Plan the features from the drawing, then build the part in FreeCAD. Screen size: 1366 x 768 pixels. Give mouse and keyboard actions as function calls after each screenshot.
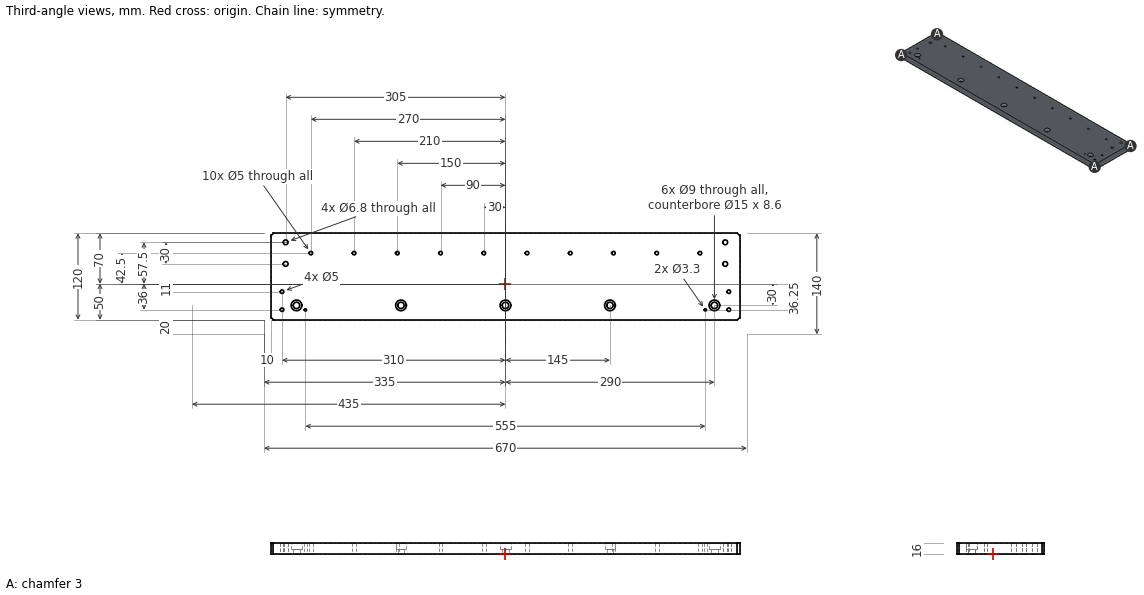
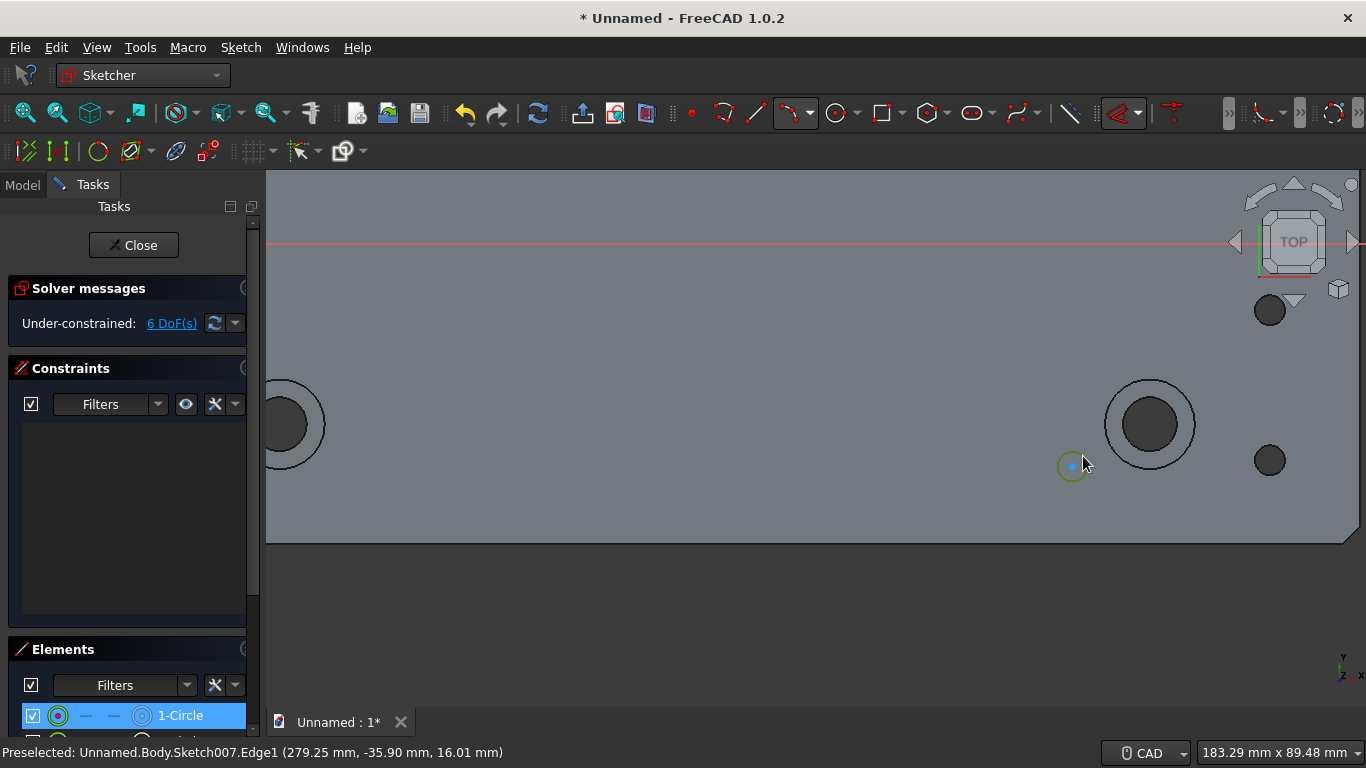
scroll(1086, 459, down, 8)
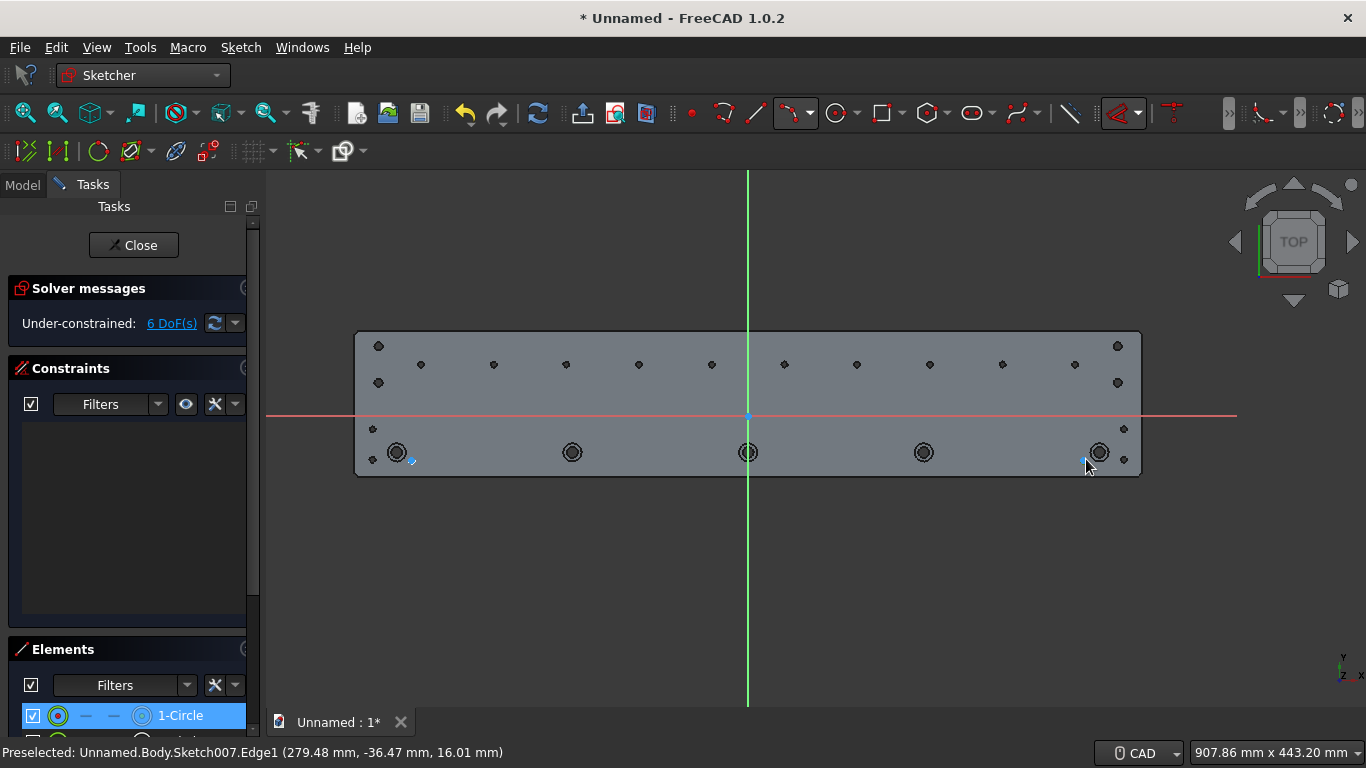
scroll(414, 459, up, 9)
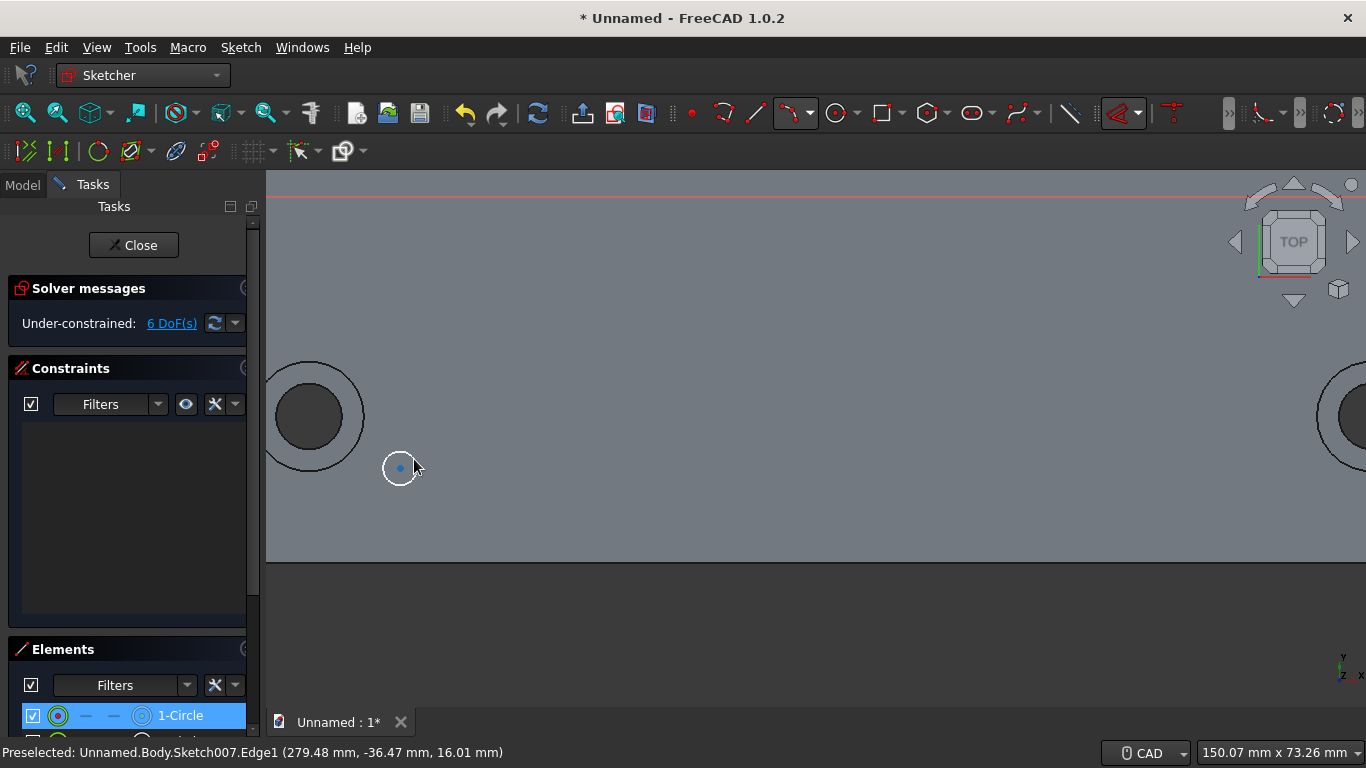
click(412, 456)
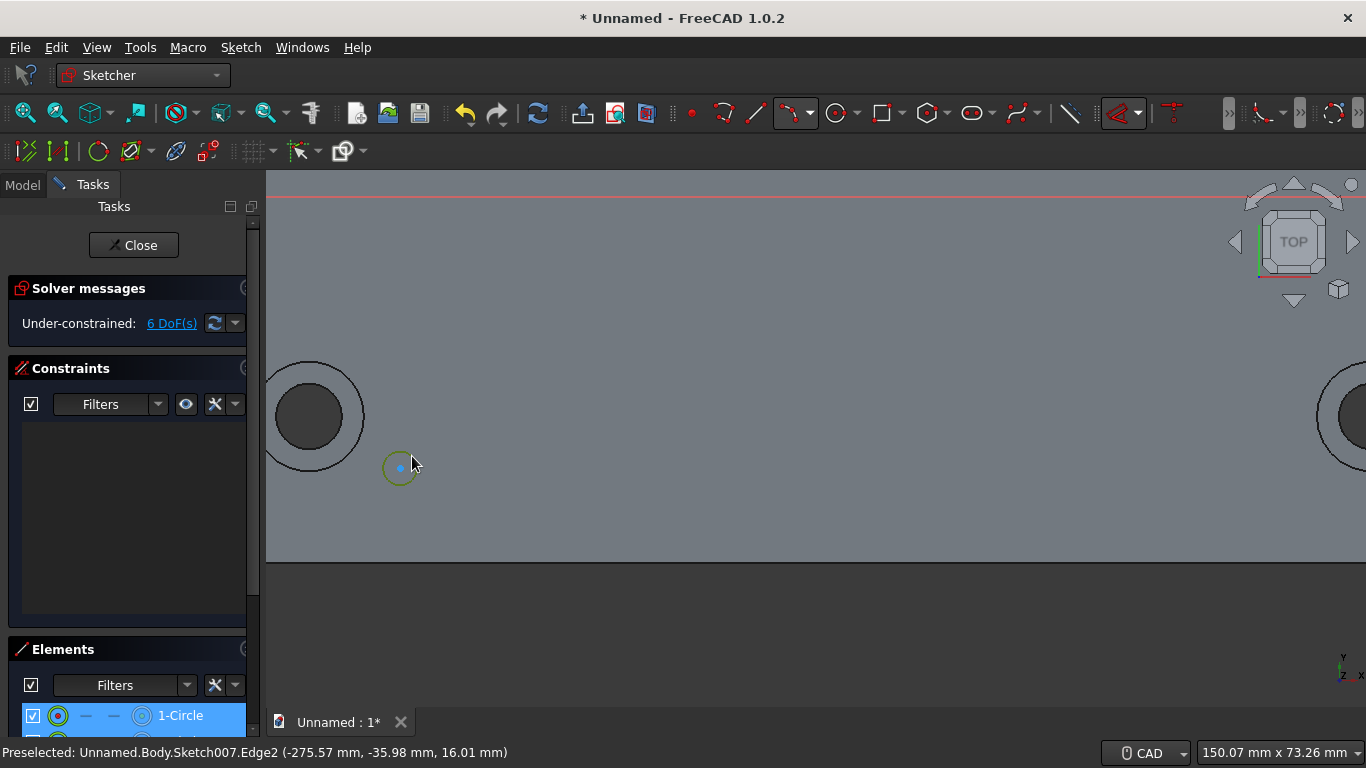
key(e)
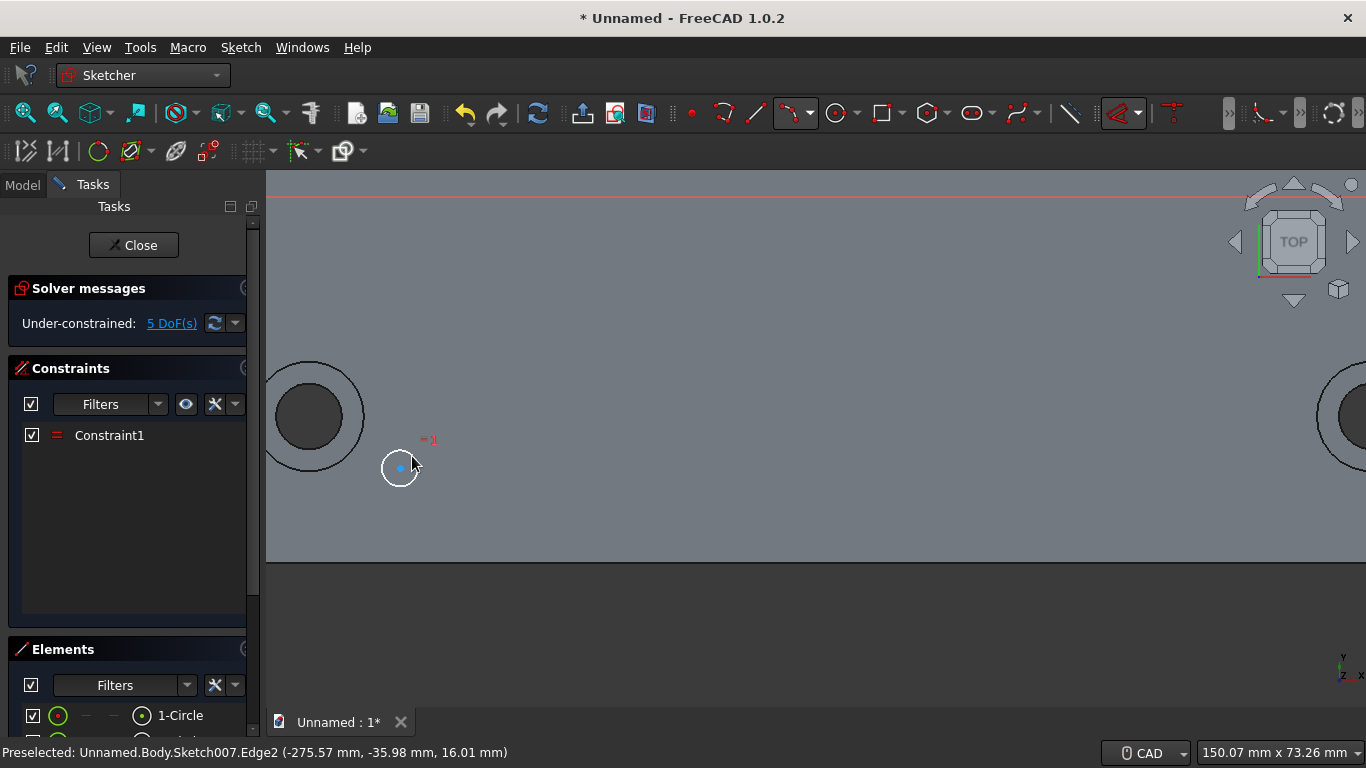
scroll(413, 459, down, 9)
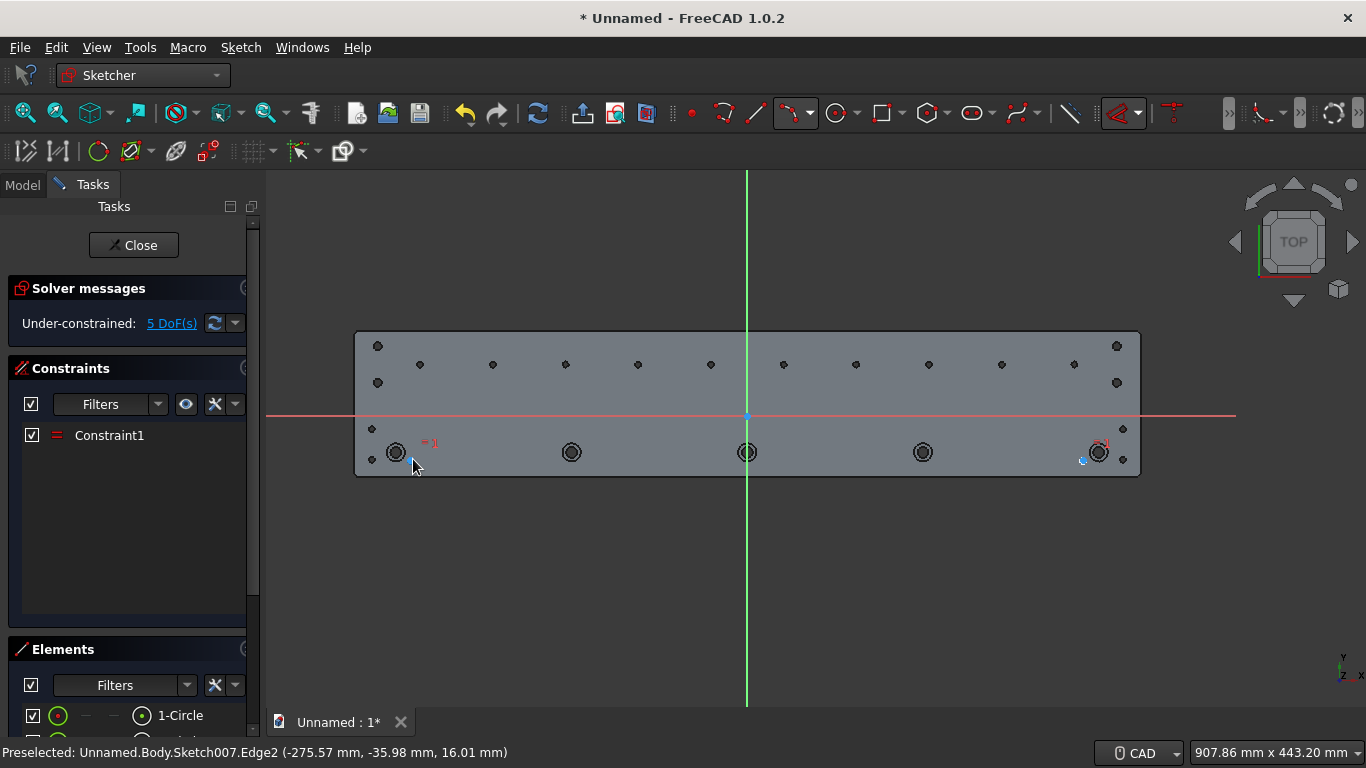
click(1083, 461)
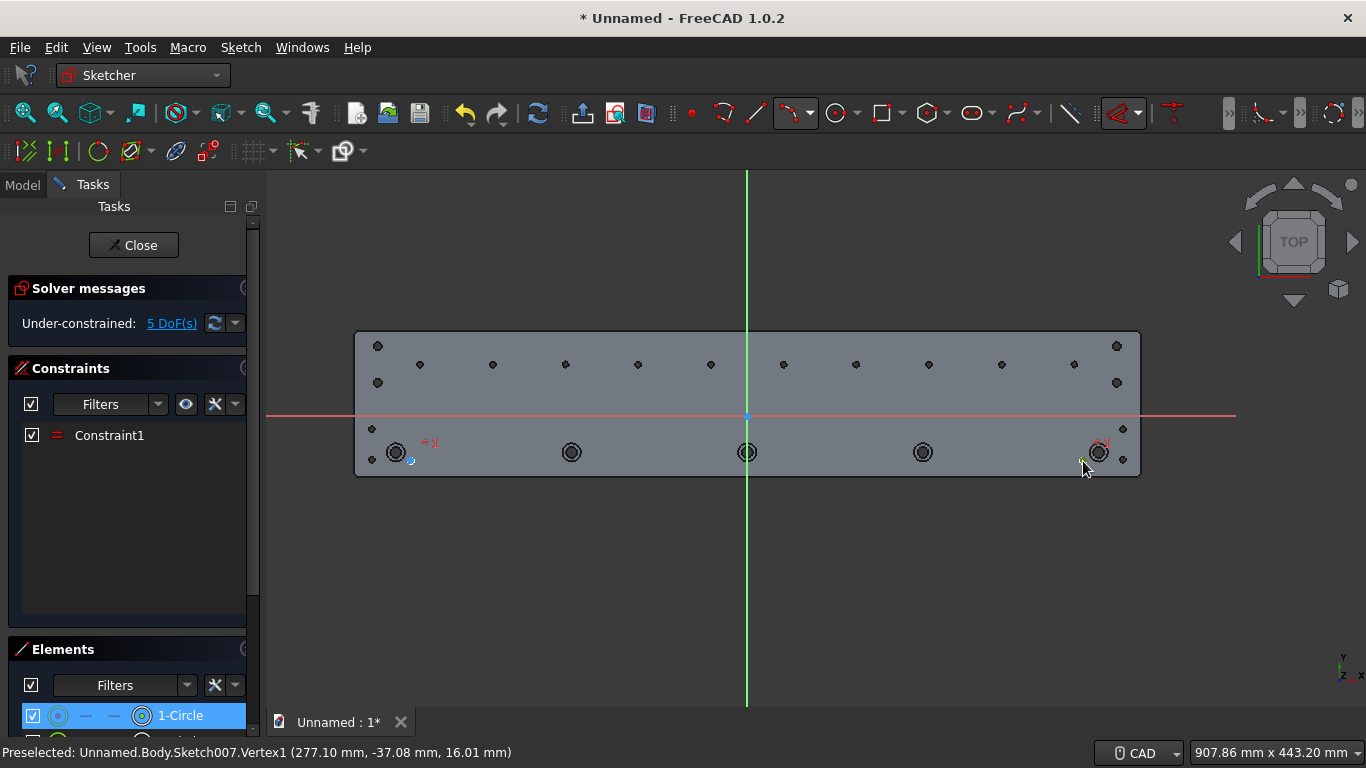
click(411, 461)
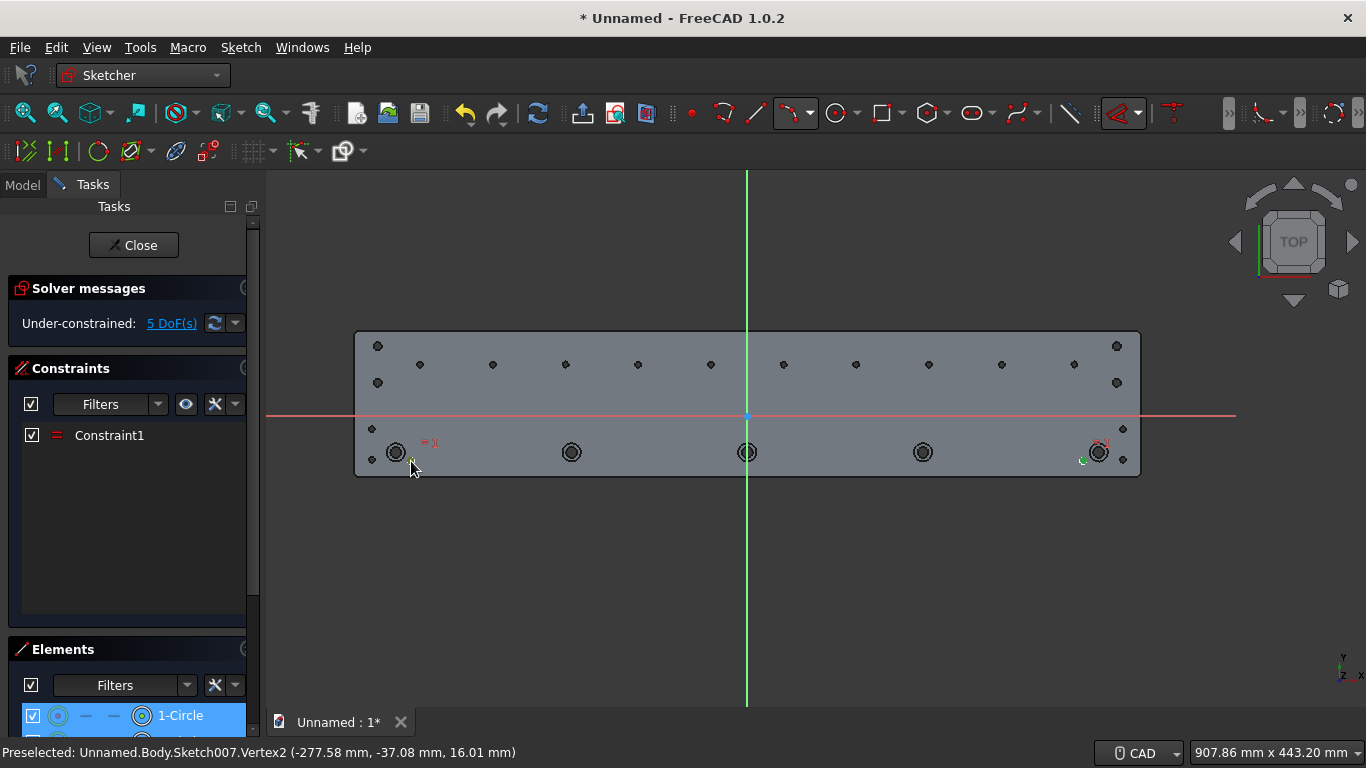
click(747, 645)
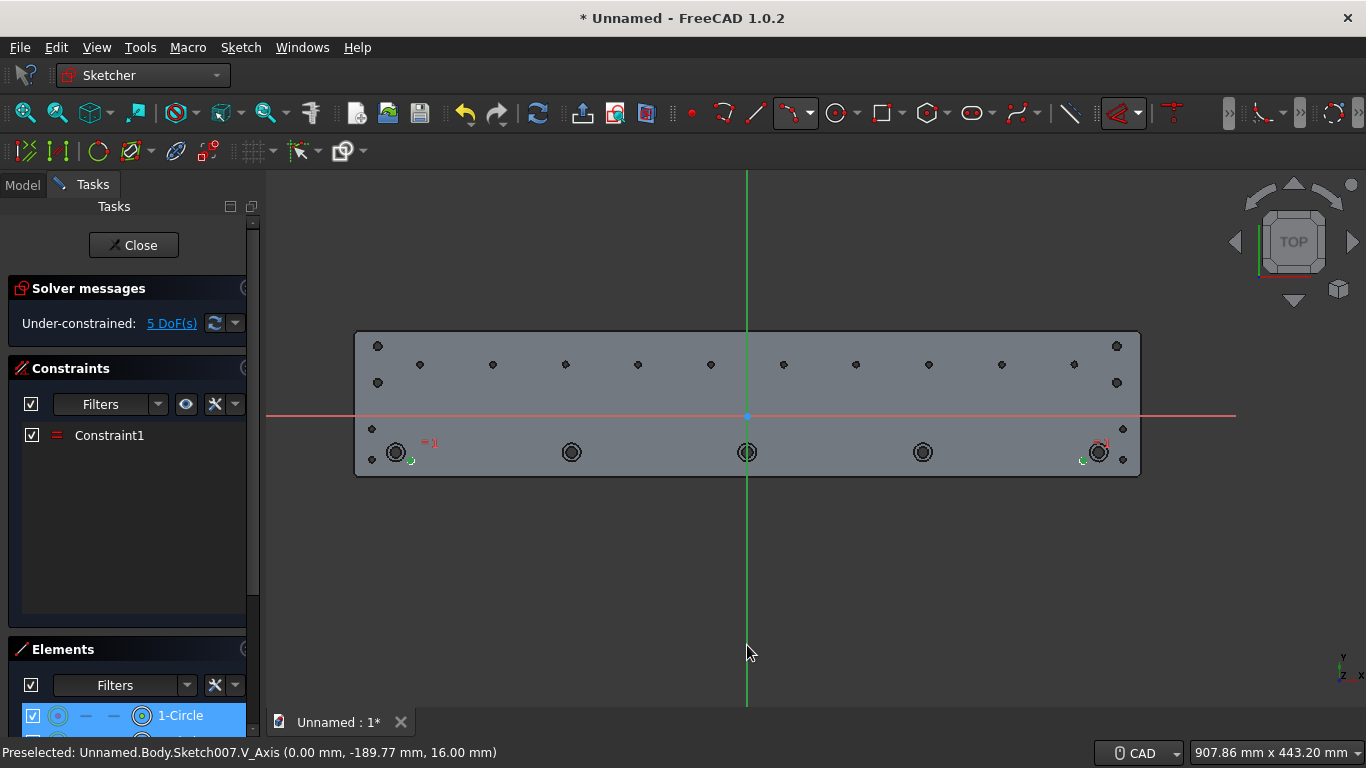
key(s)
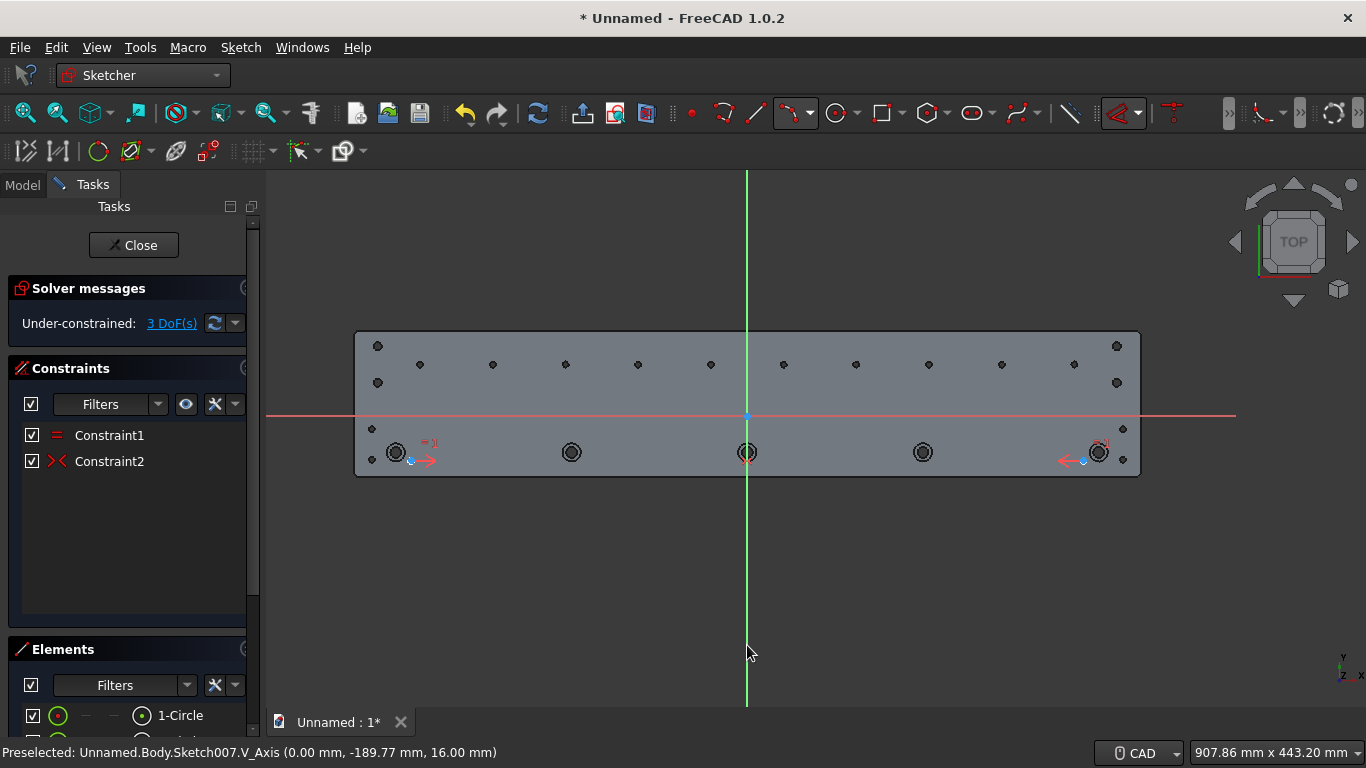
scroll(1081, 459, up, 12)